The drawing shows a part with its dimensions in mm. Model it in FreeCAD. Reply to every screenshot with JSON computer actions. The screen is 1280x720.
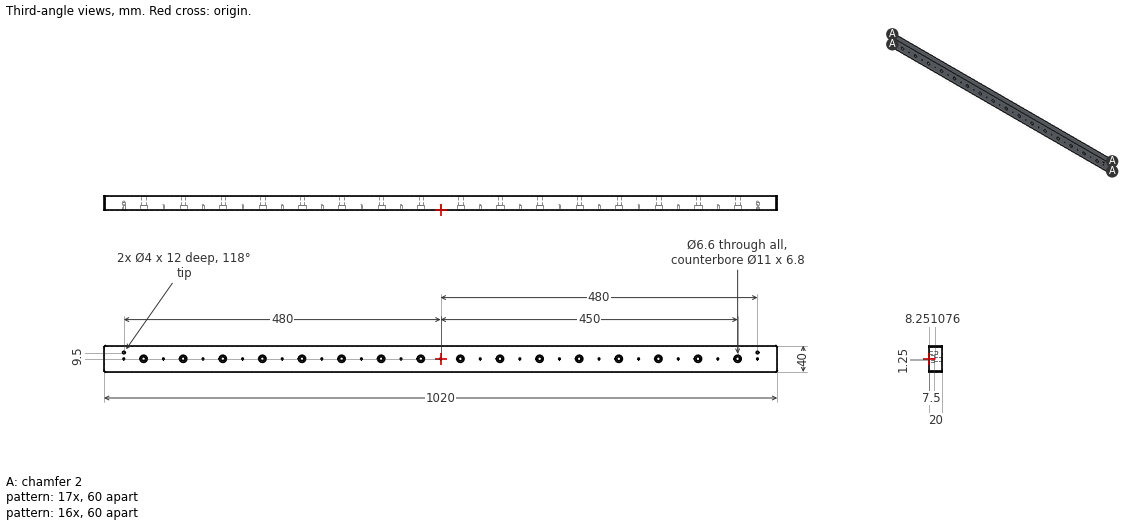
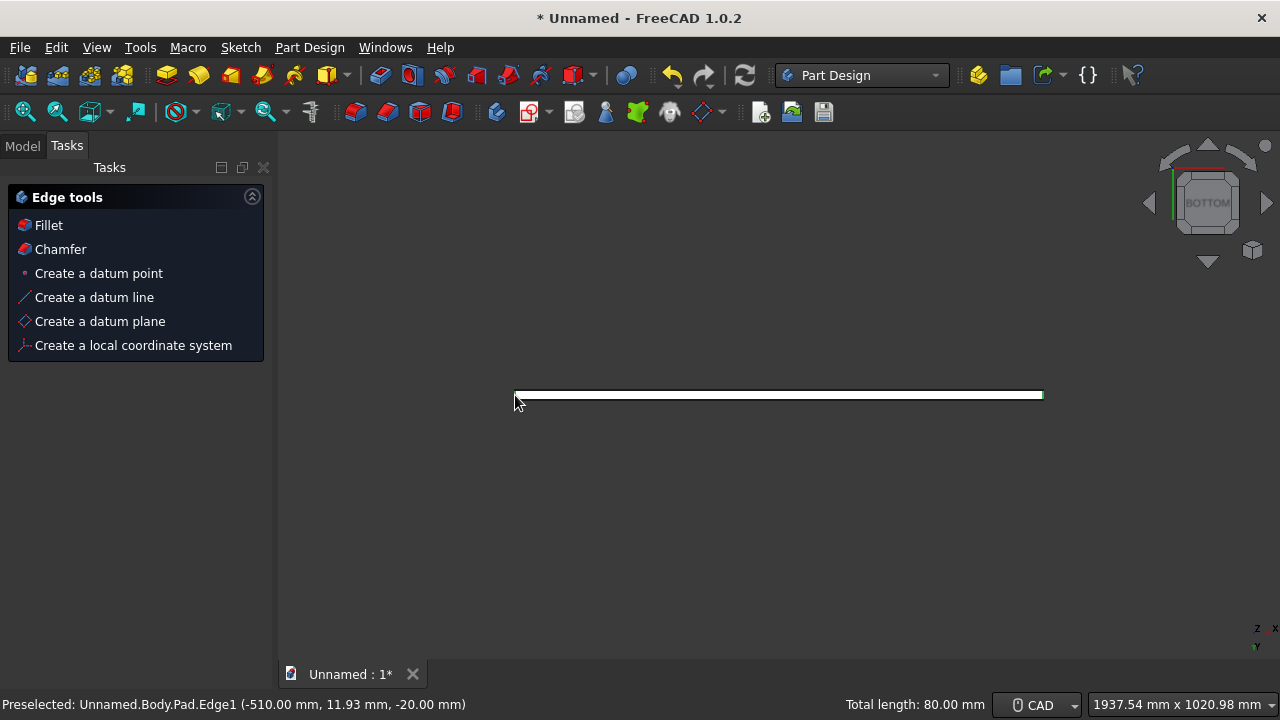
{"action": "left_click", "coordinate": [388, 112]}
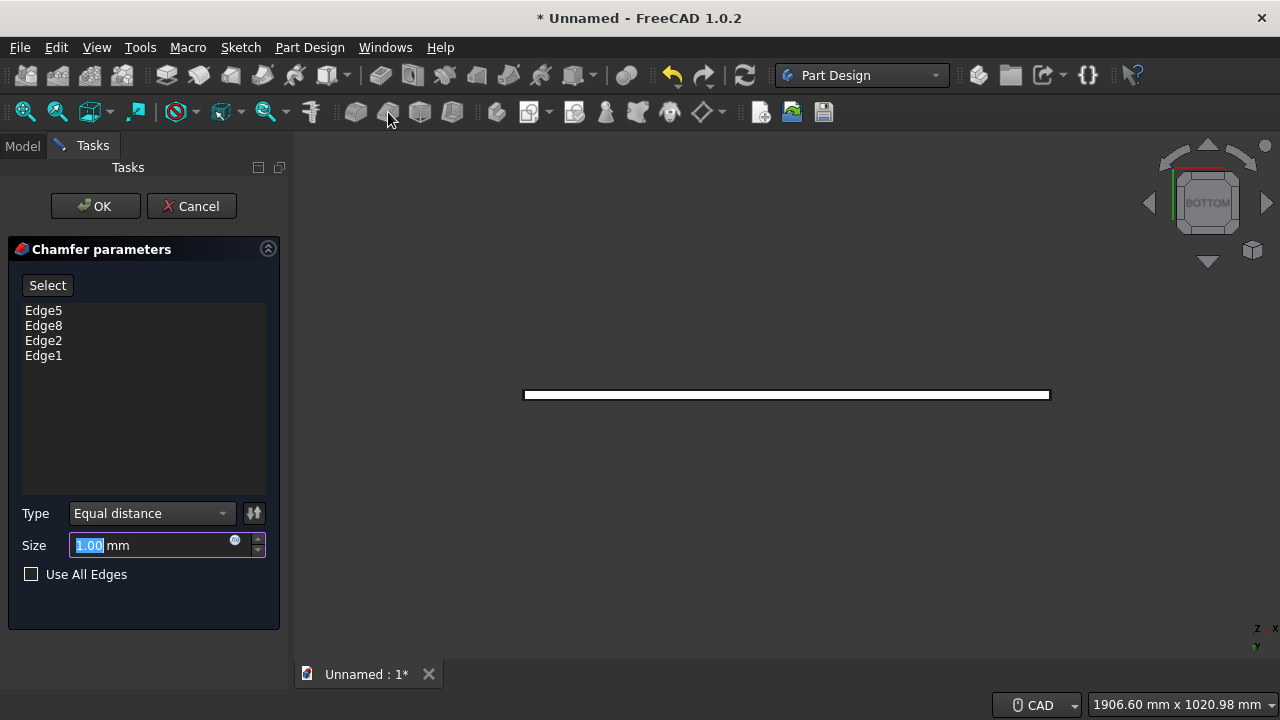
{"action": "type", "text": "2"}
{"action": "key", "text": "Tab"}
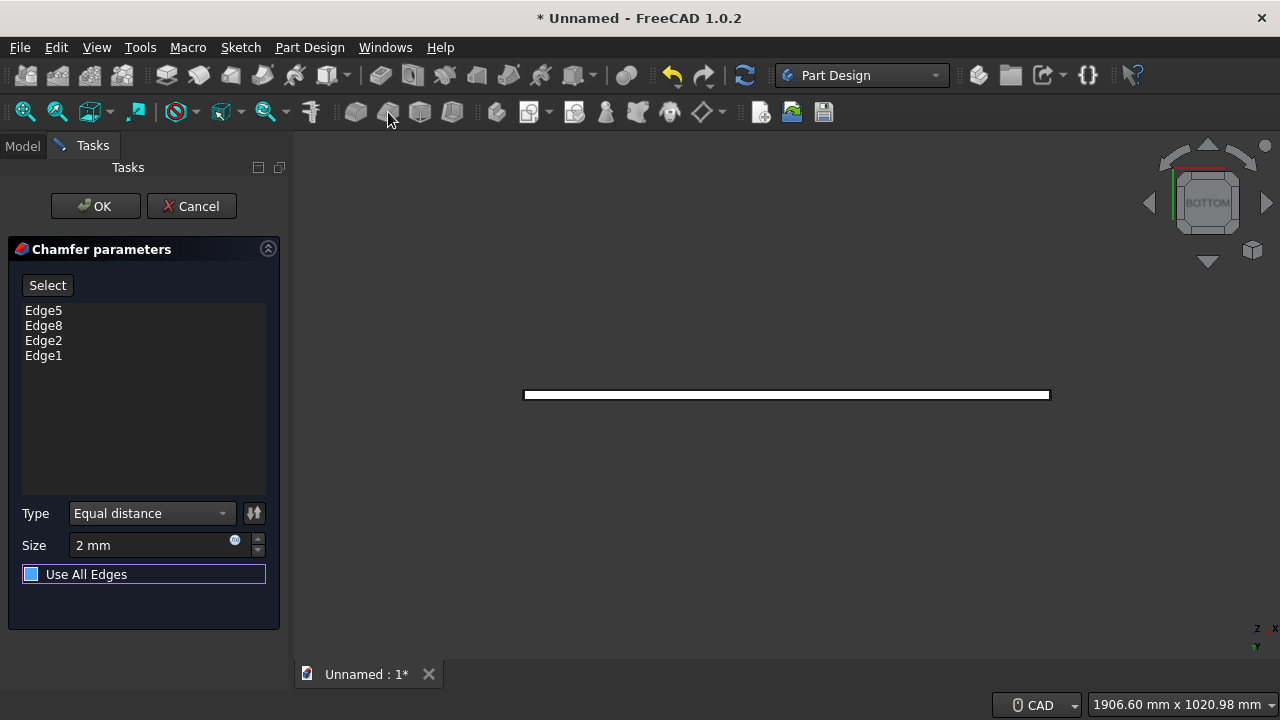
{"action": "left_click", "coordinate": [96, 206]}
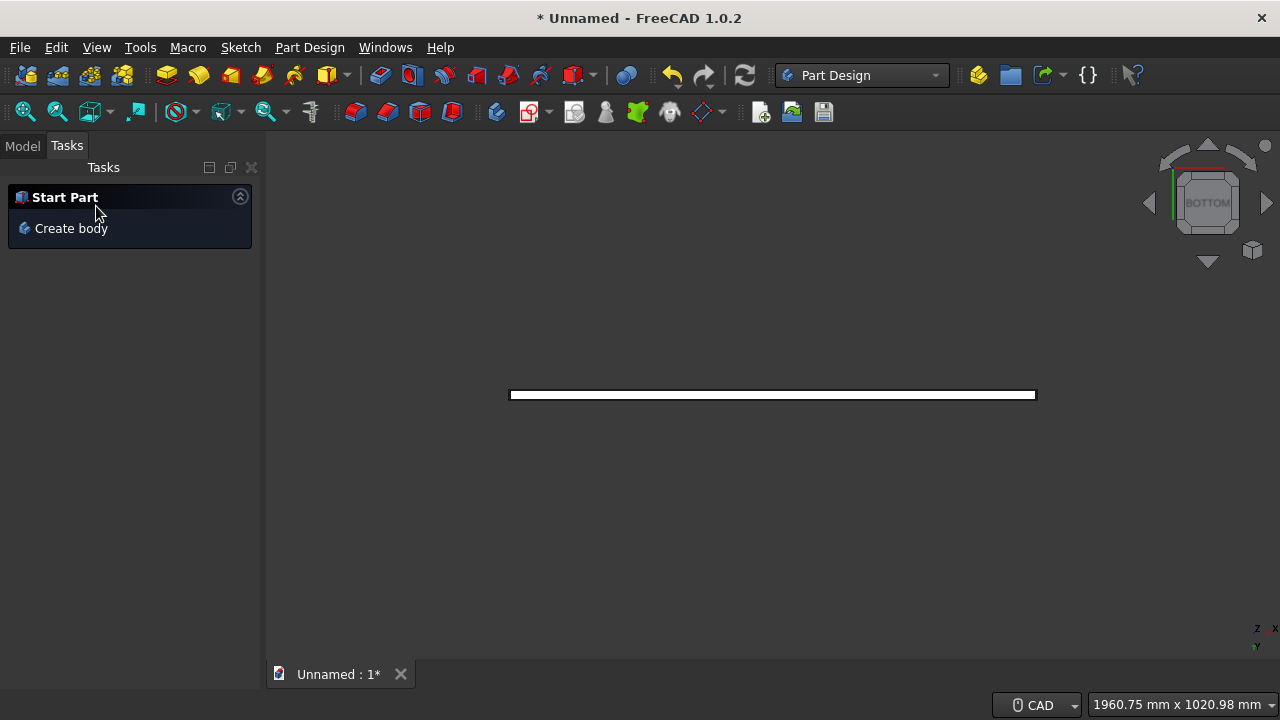
{"action": "key", "text": "0"}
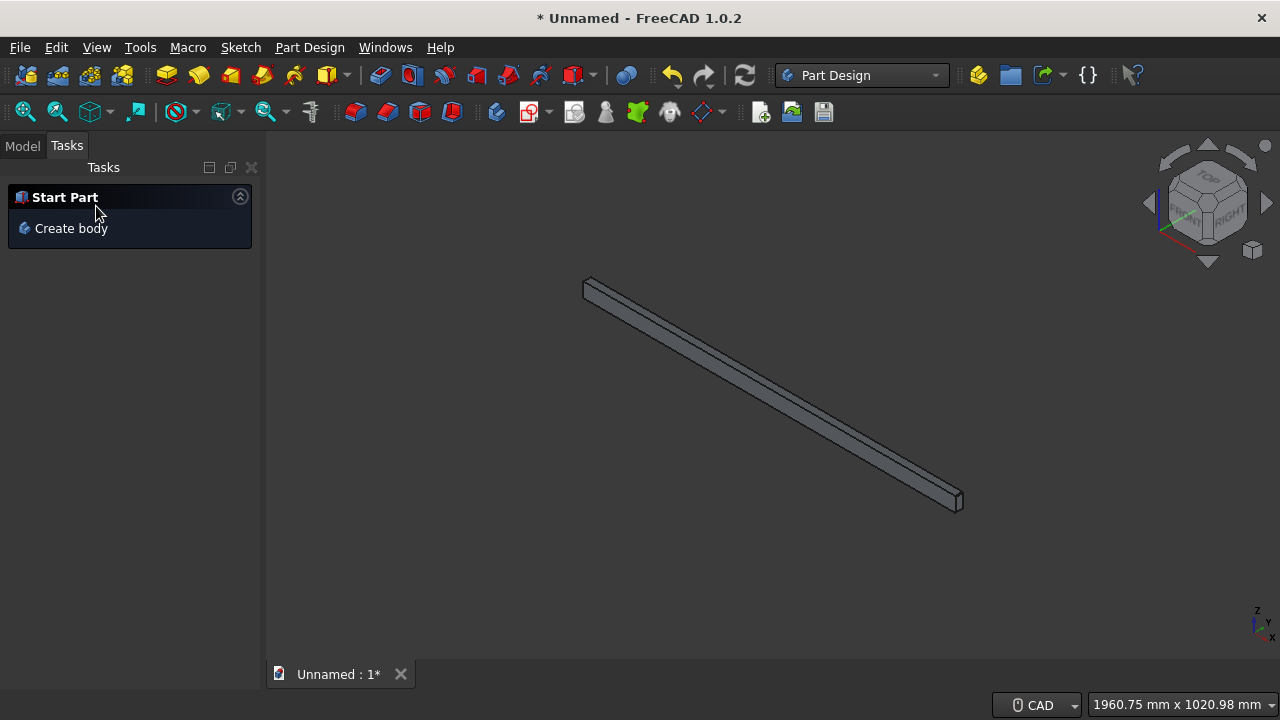
{"action": "key", "text": "v f"}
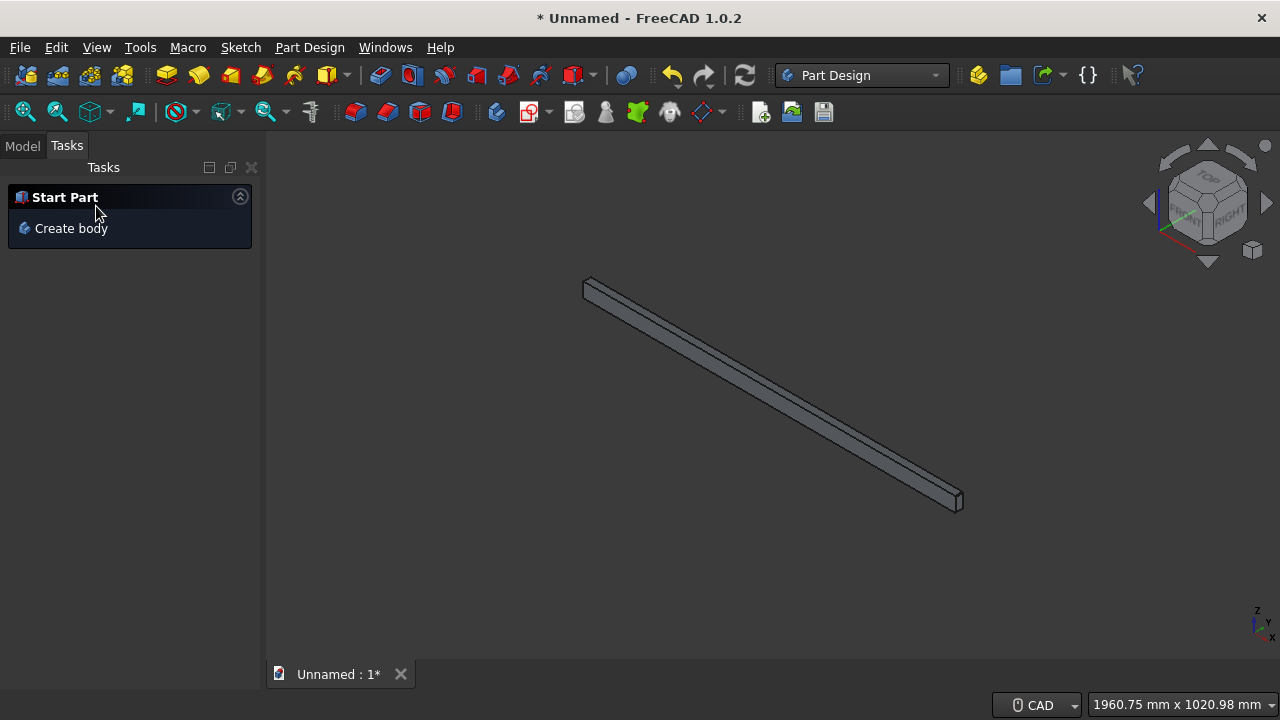
{"action": "key", "text": "1"}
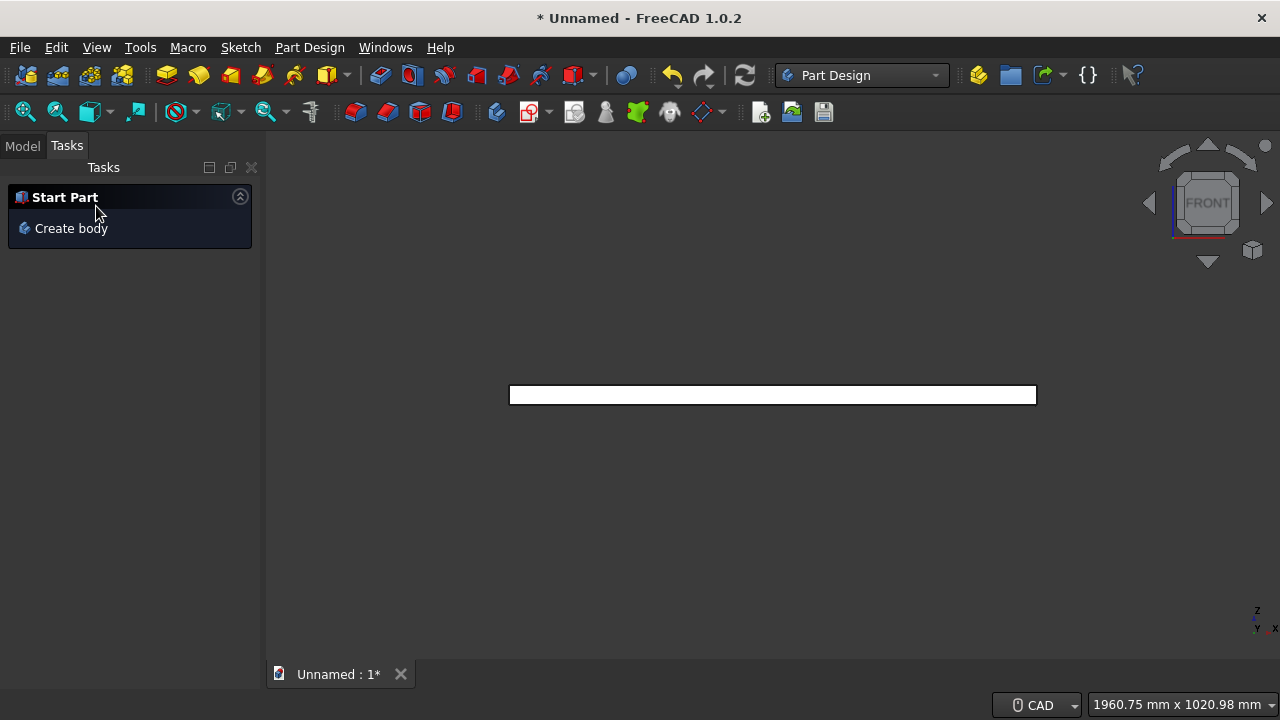
{"action": "left_click", "coordinate": [999, 394]}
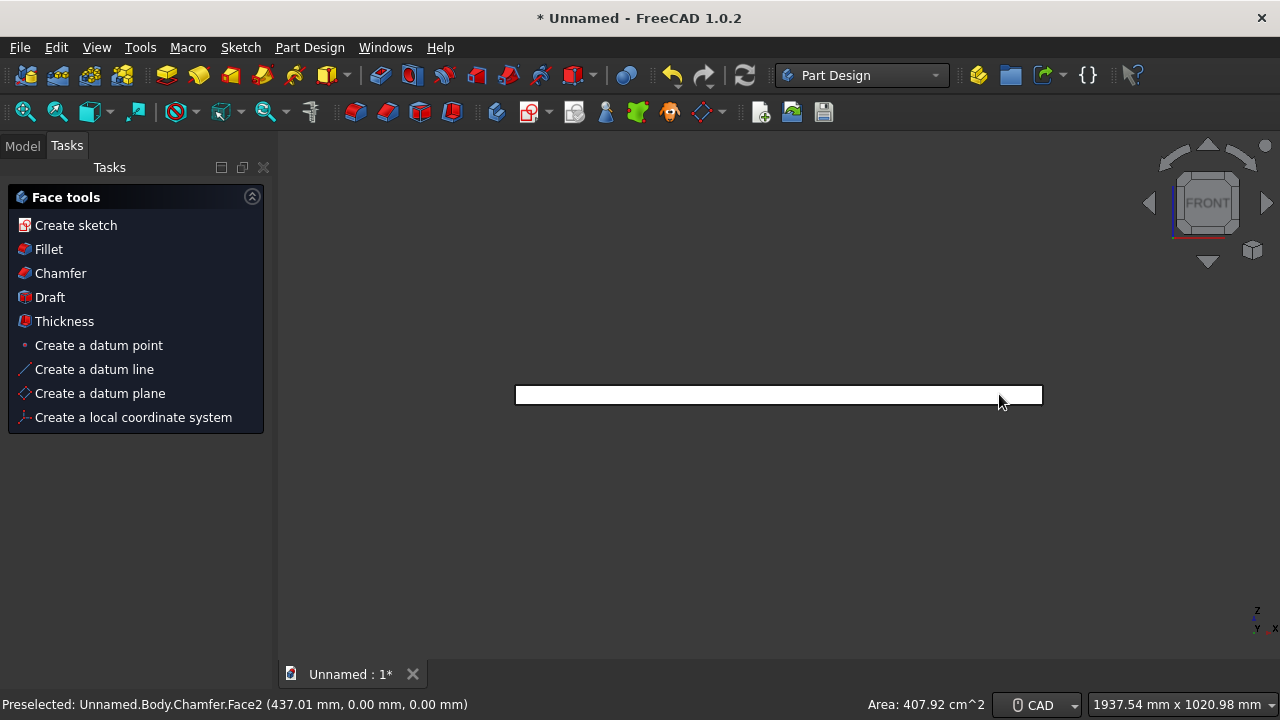
{"action": "left_click", "coordinate": [530, 112]}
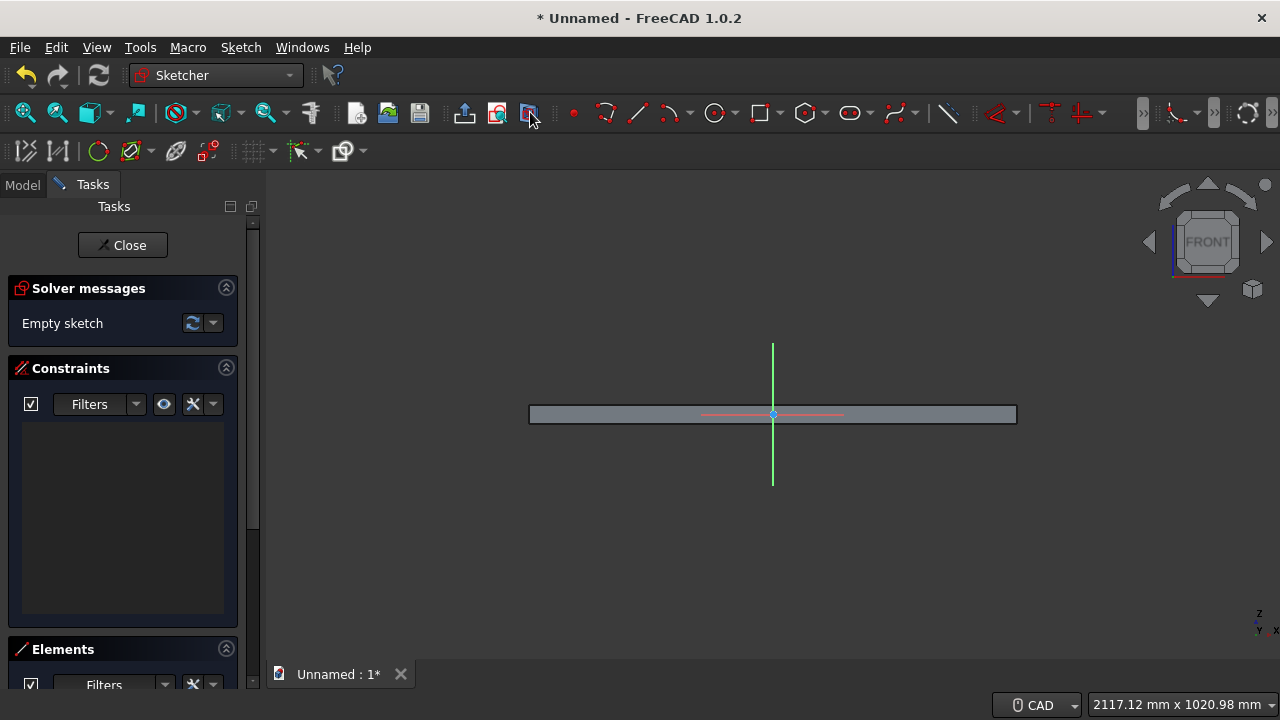
{"action": "key", "text": "g c"}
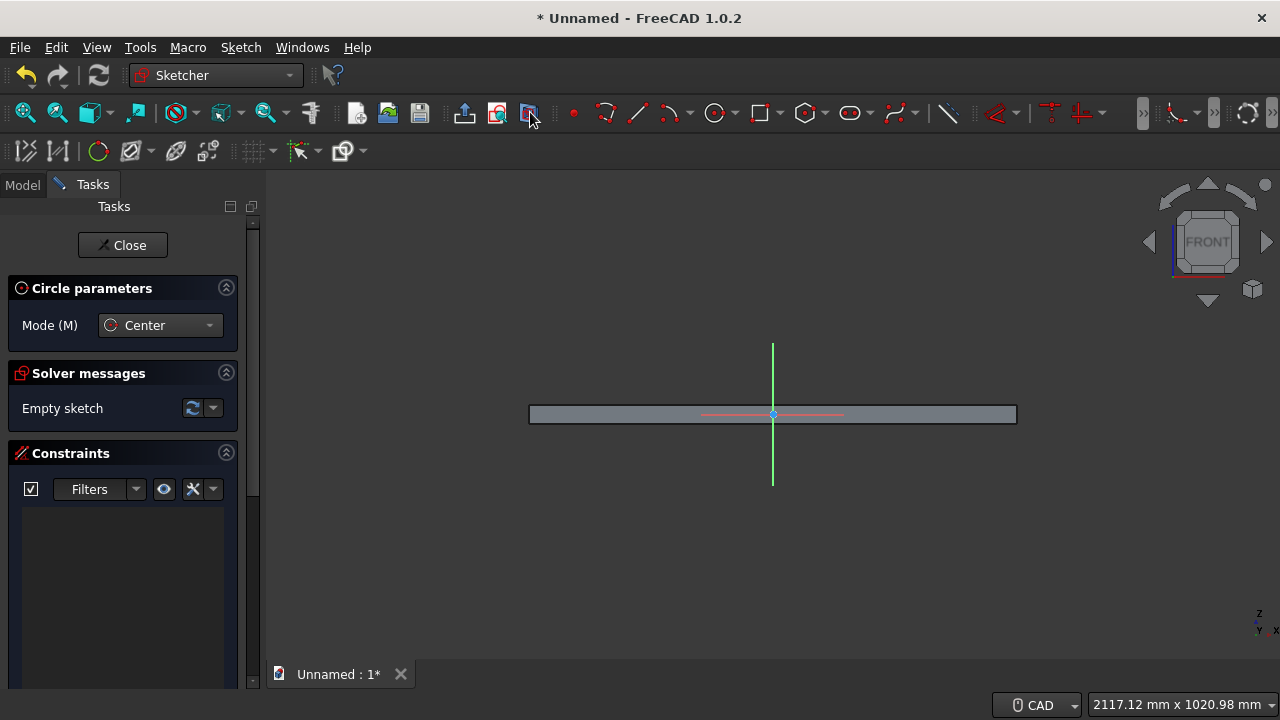
{"action": "scroll", "coordinate": [543, 410], "scroll_direction": "up", "scroll_amount": 16}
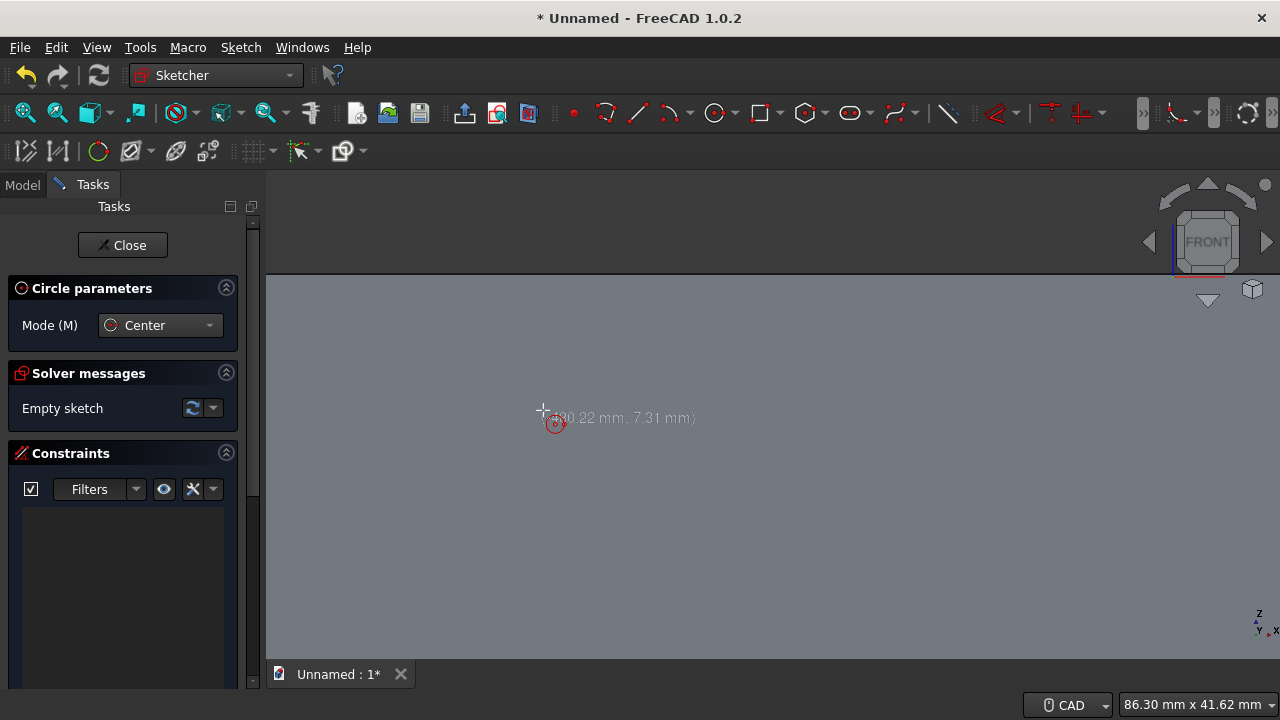
{"action": "scroll", "coordinate": [418, 413], "scroll_direction": "down", "scroll_amount": 15}